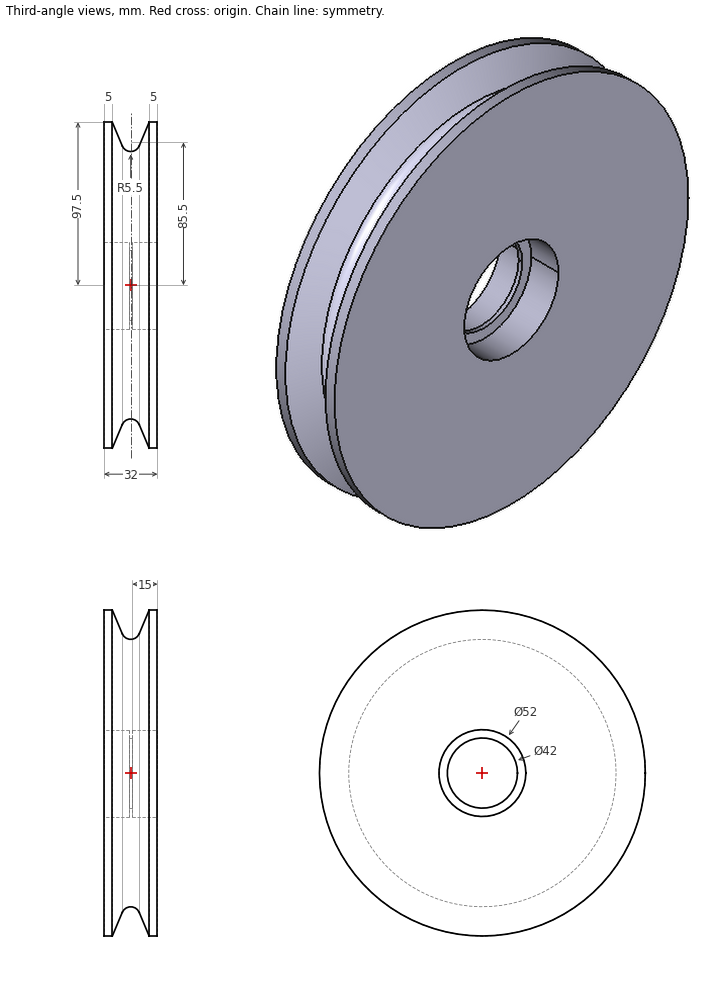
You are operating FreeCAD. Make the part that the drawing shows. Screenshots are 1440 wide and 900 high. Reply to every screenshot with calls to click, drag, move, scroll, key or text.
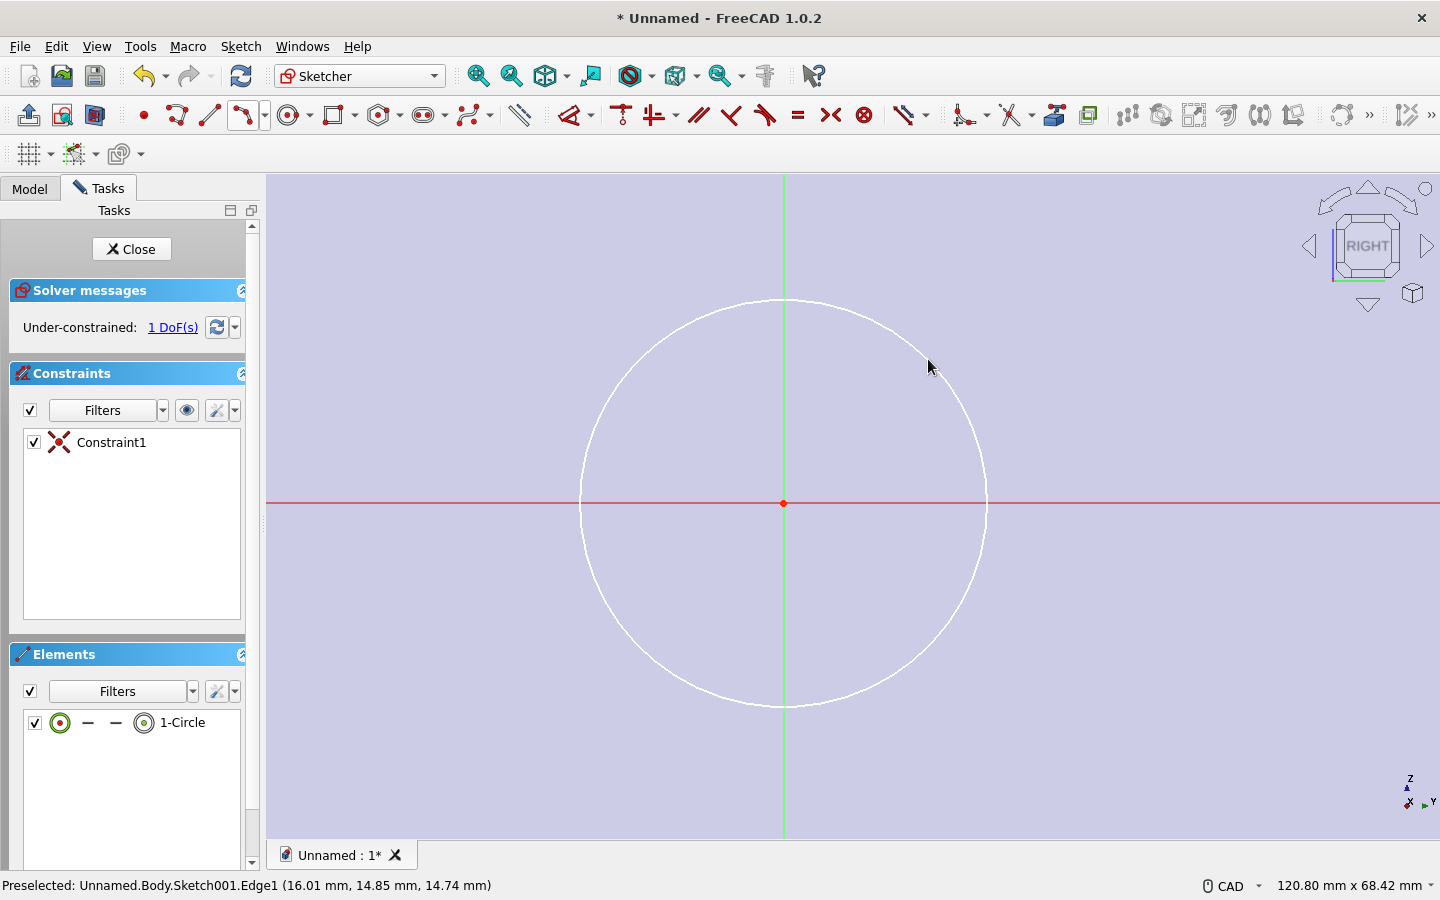
click(568, 116)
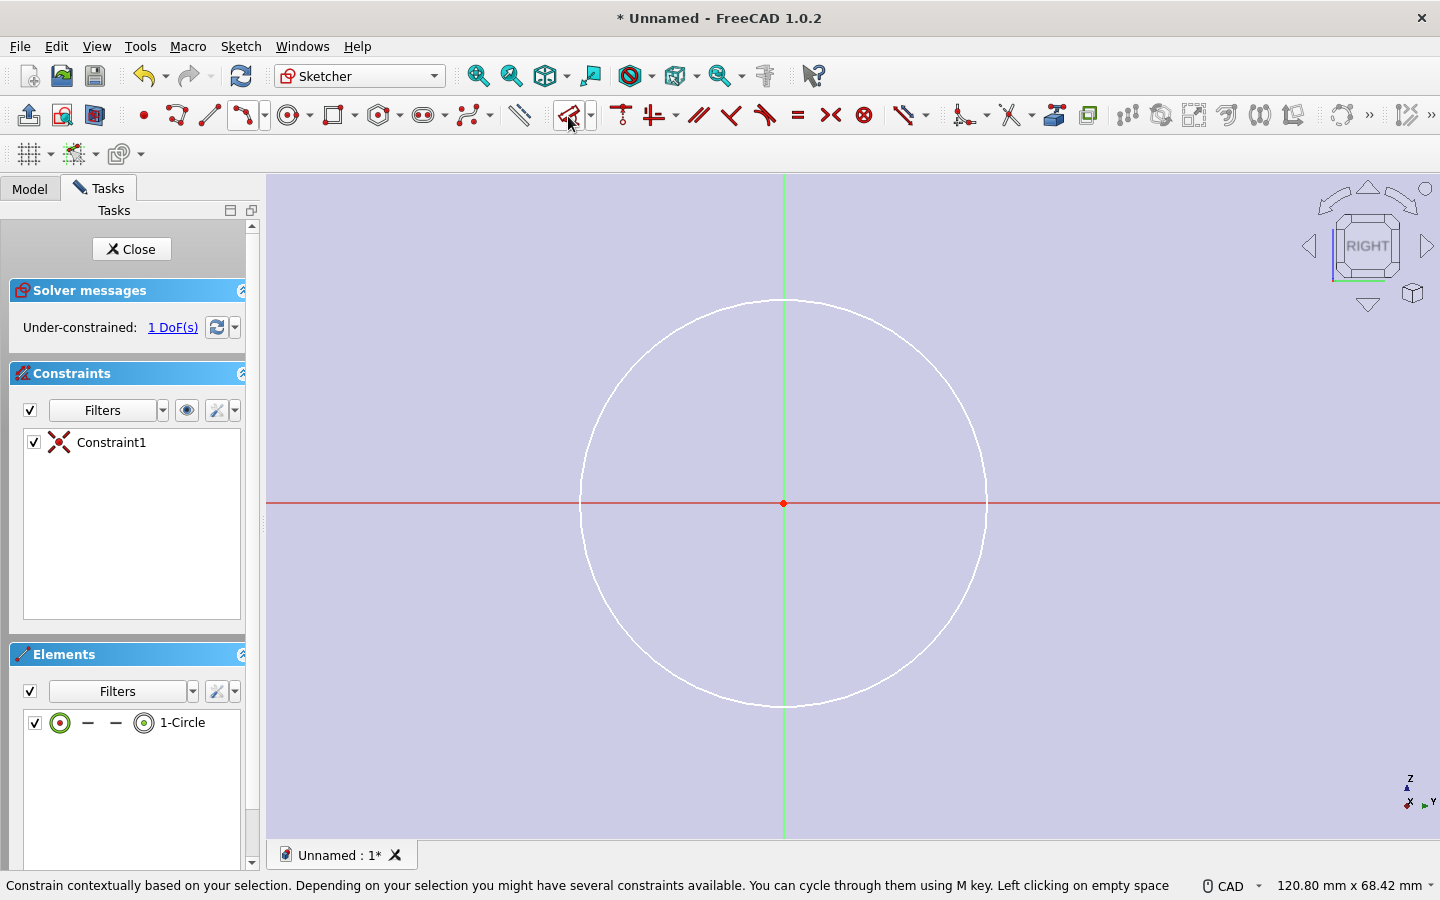
click(927, 359)
click(950, 336)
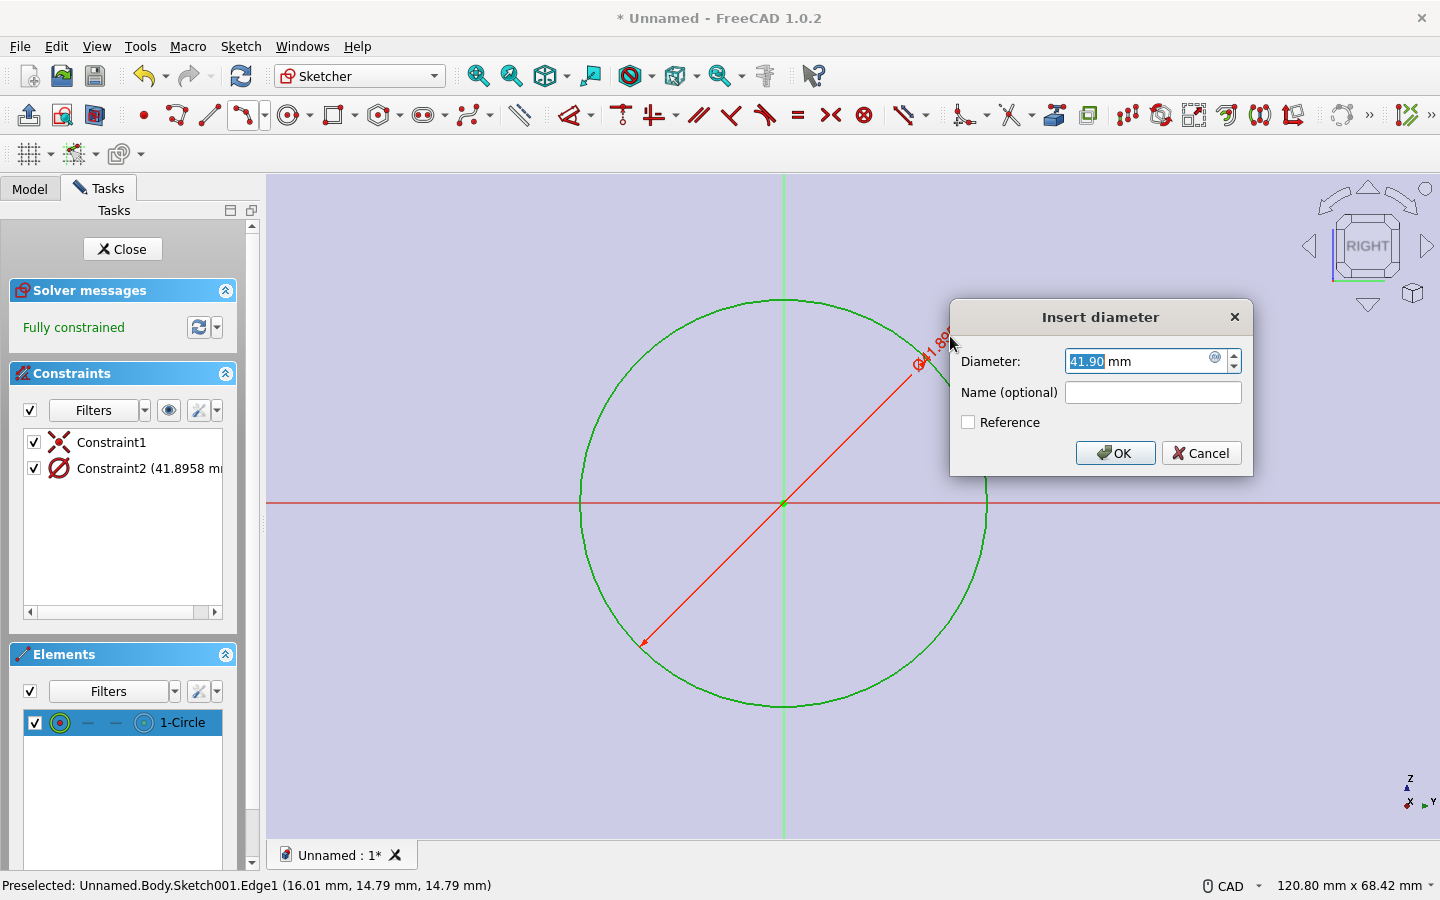
text(42)
key(Return)
key(Escape)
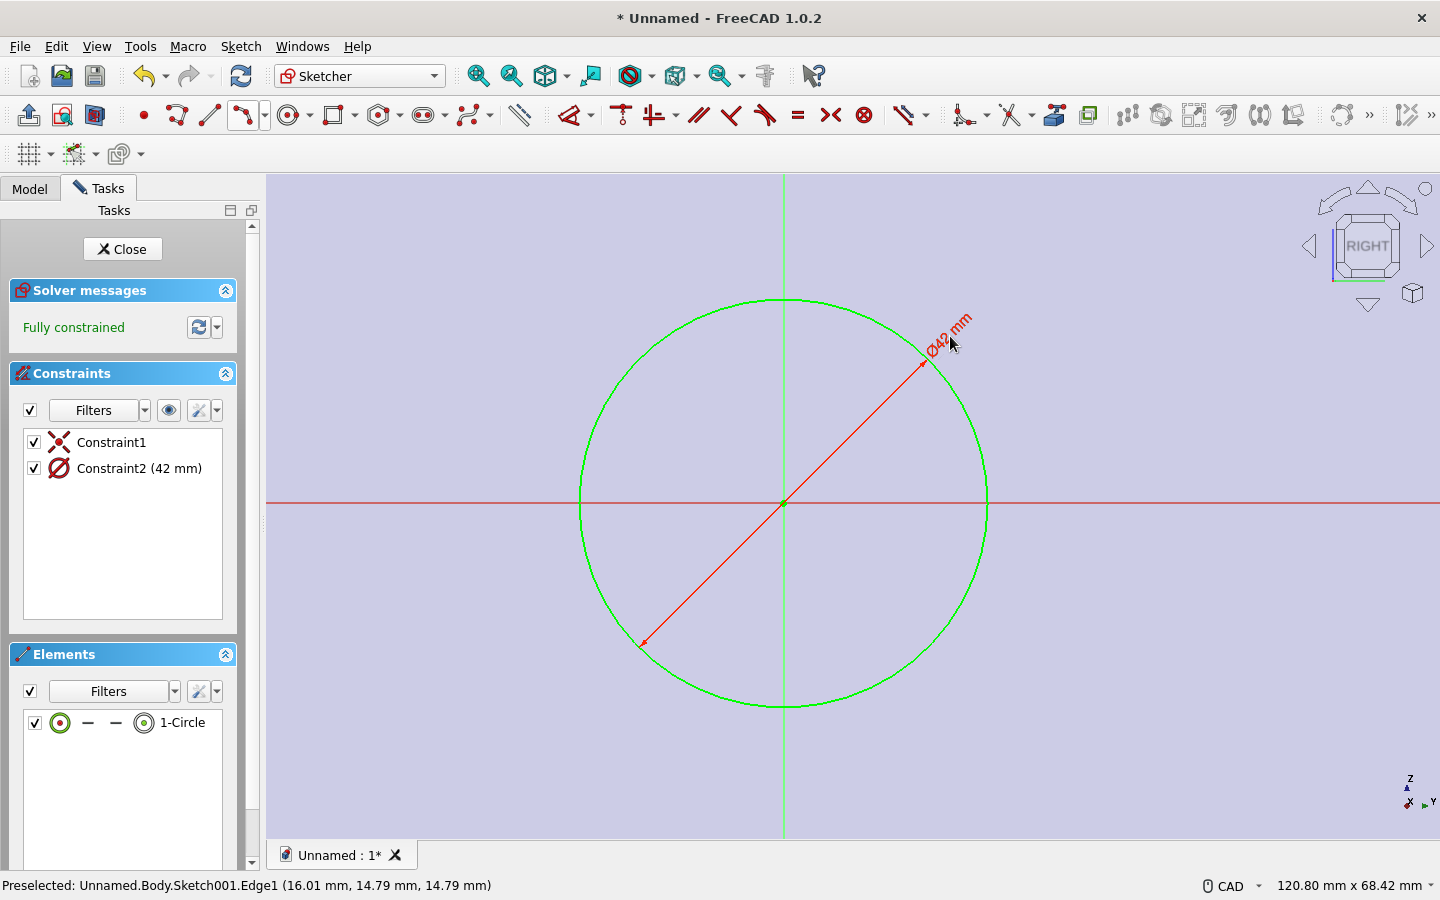
click(123, 249)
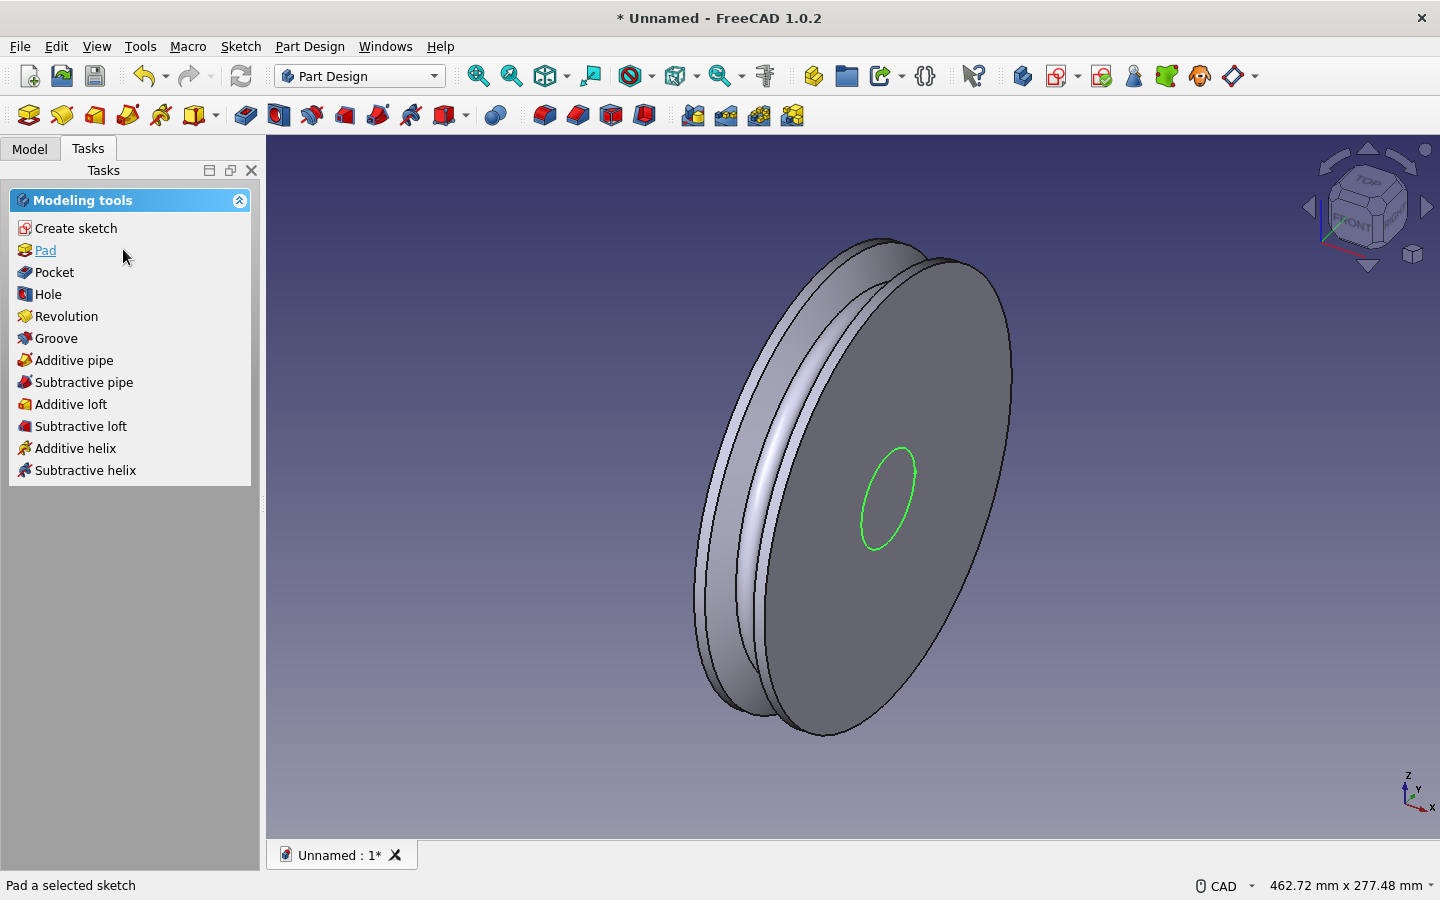
click(246, 116)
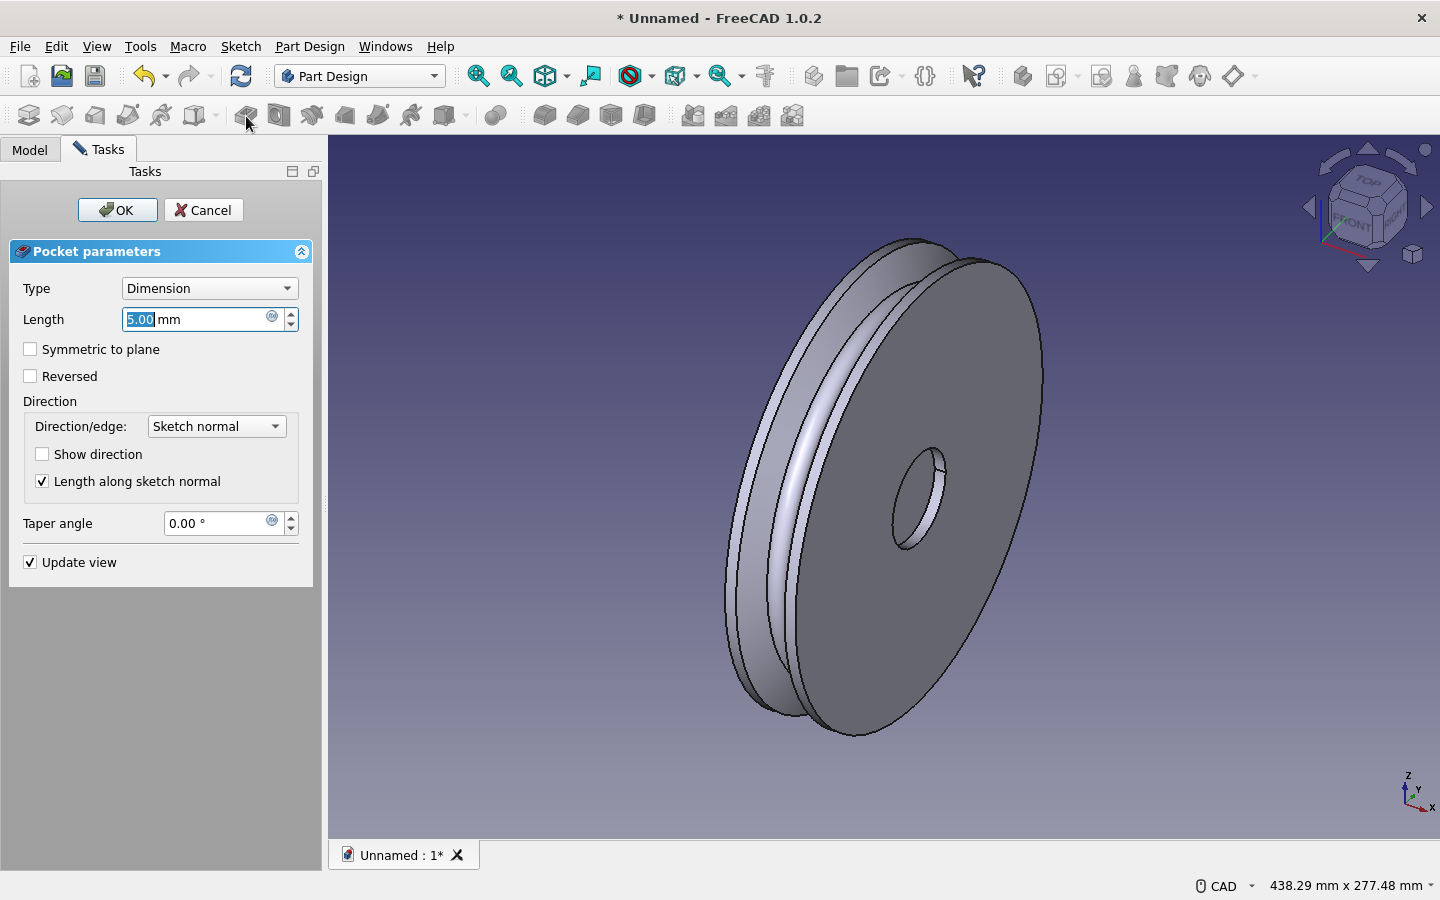
click(210, 288)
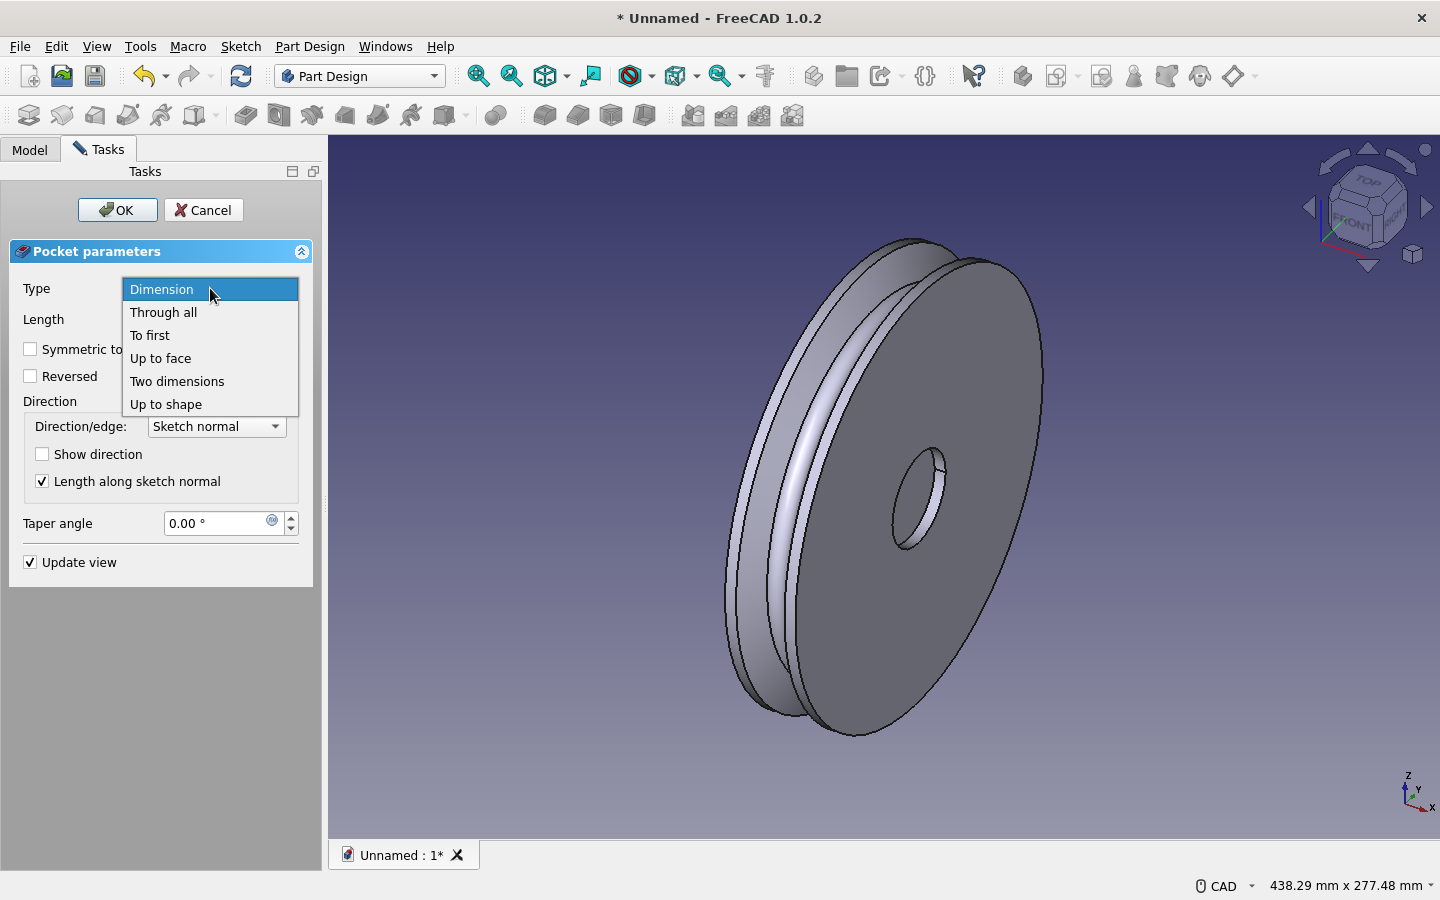
click(208, 336)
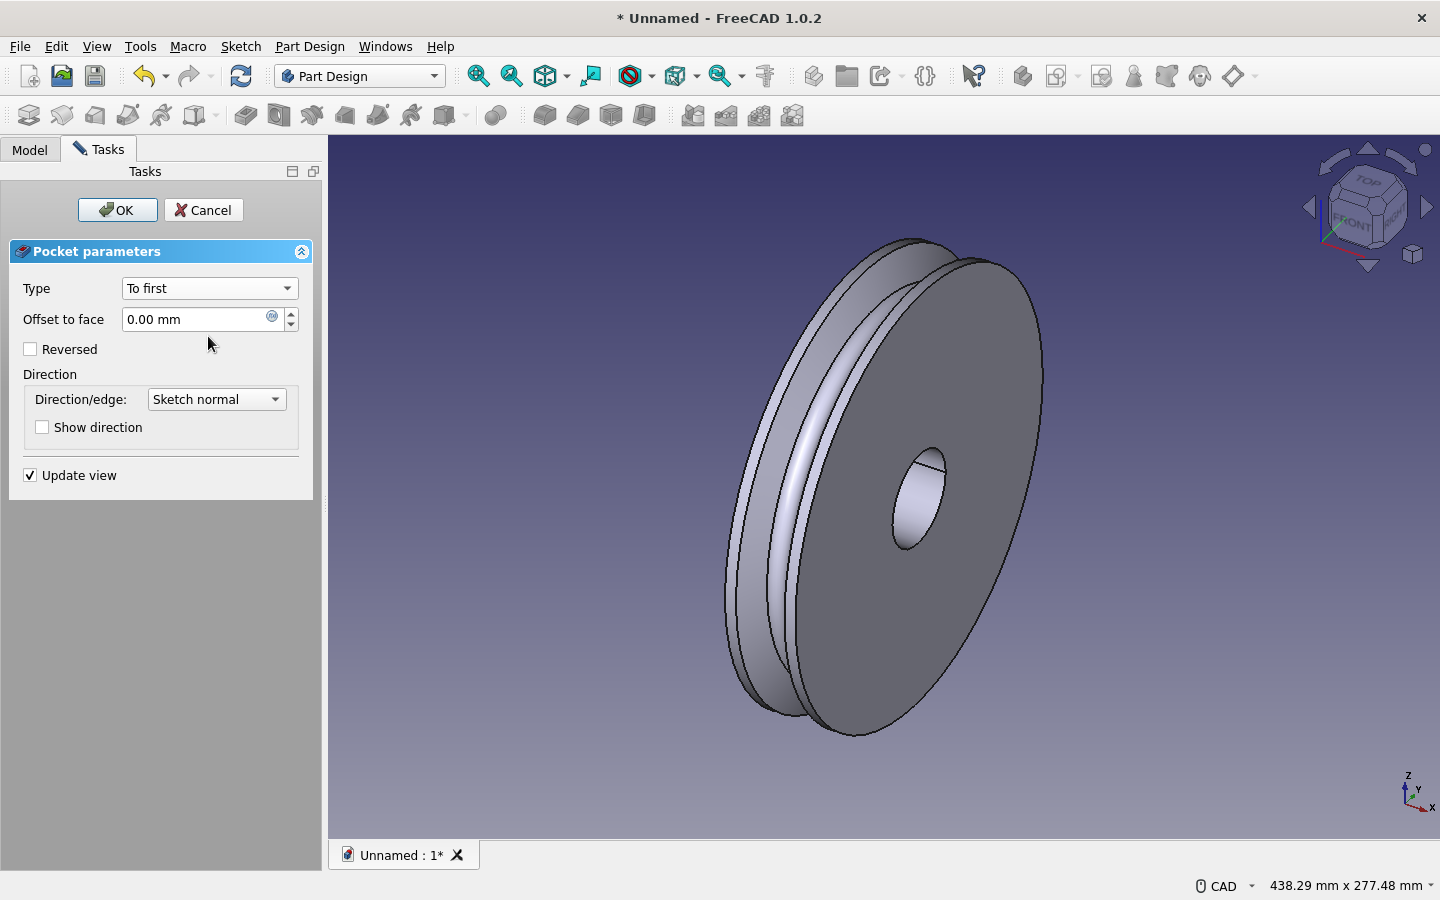
click(118, 210)